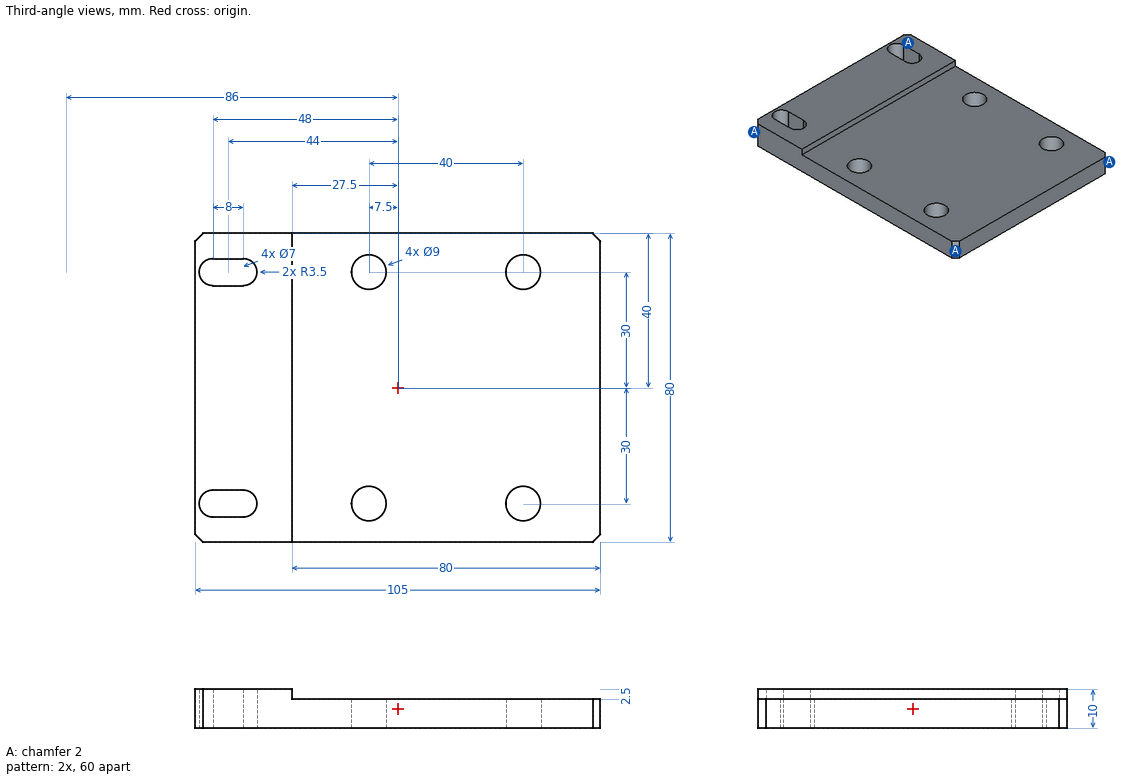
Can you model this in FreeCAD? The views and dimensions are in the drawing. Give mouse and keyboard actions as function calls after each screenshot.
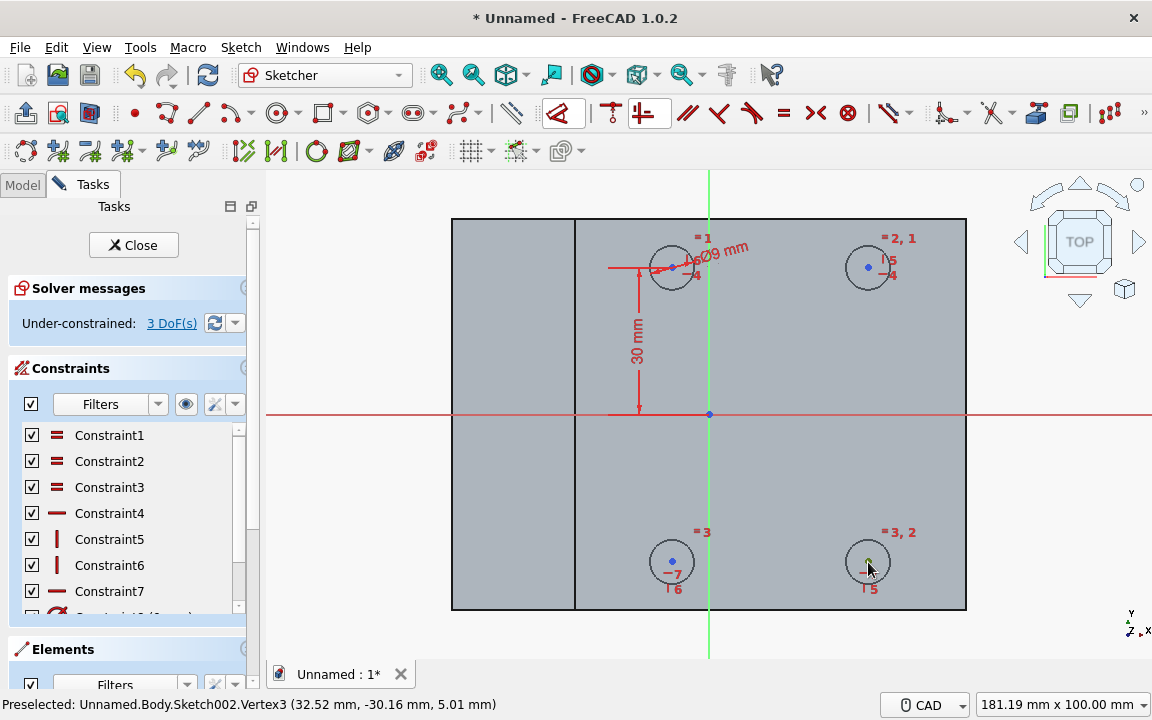
click(580, 114)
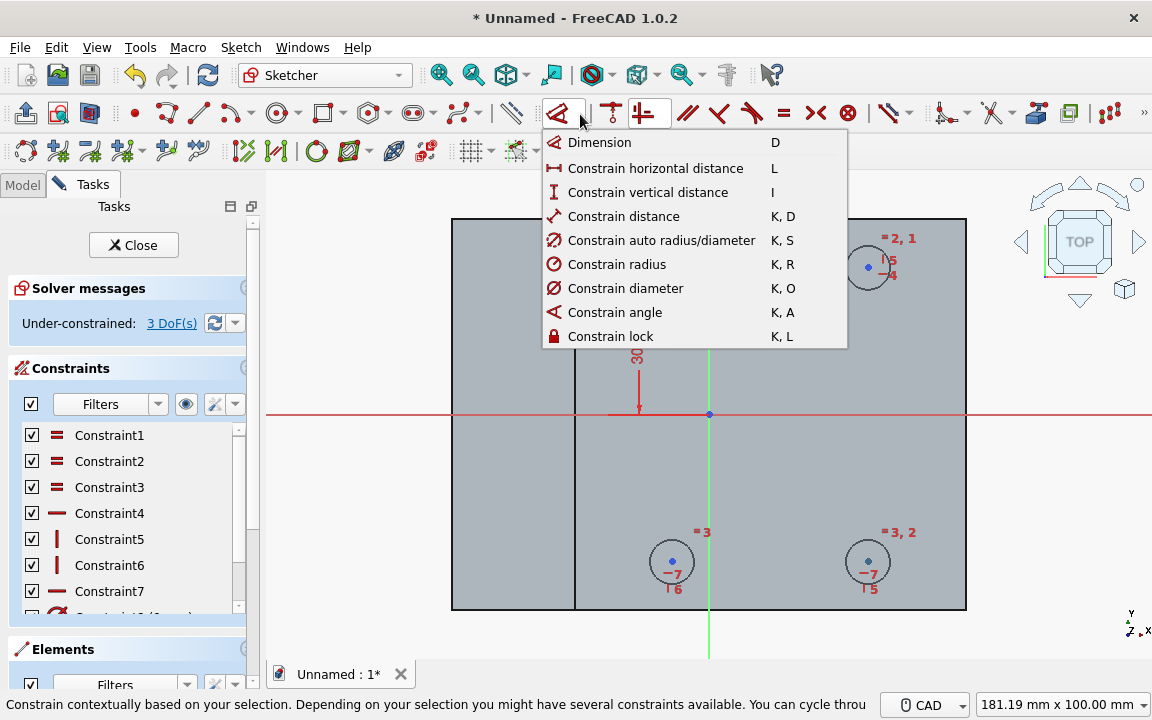
click(695, 192)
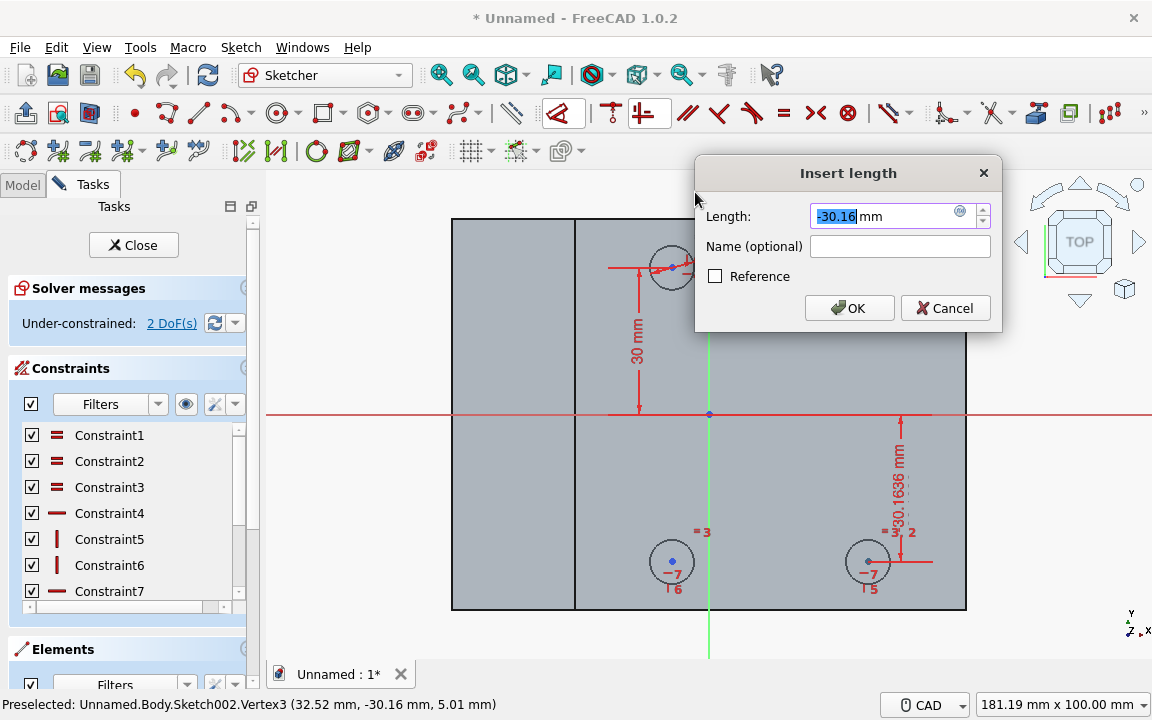
text(-30)
key(Return)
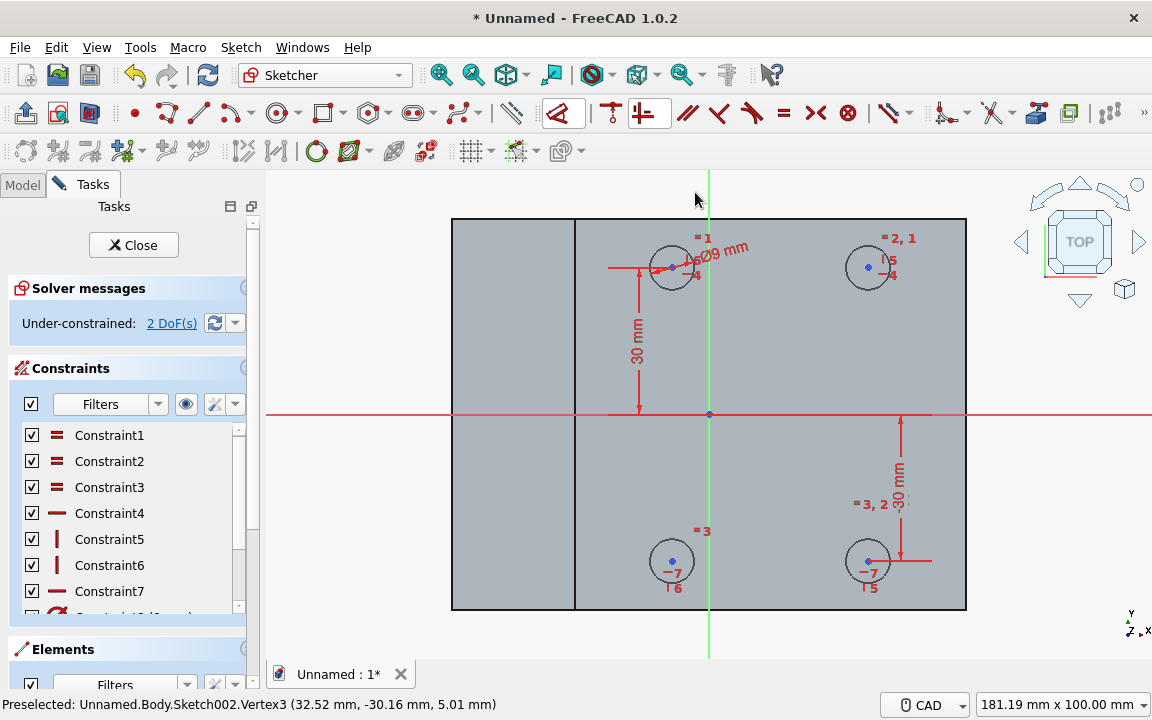
click(672, 268)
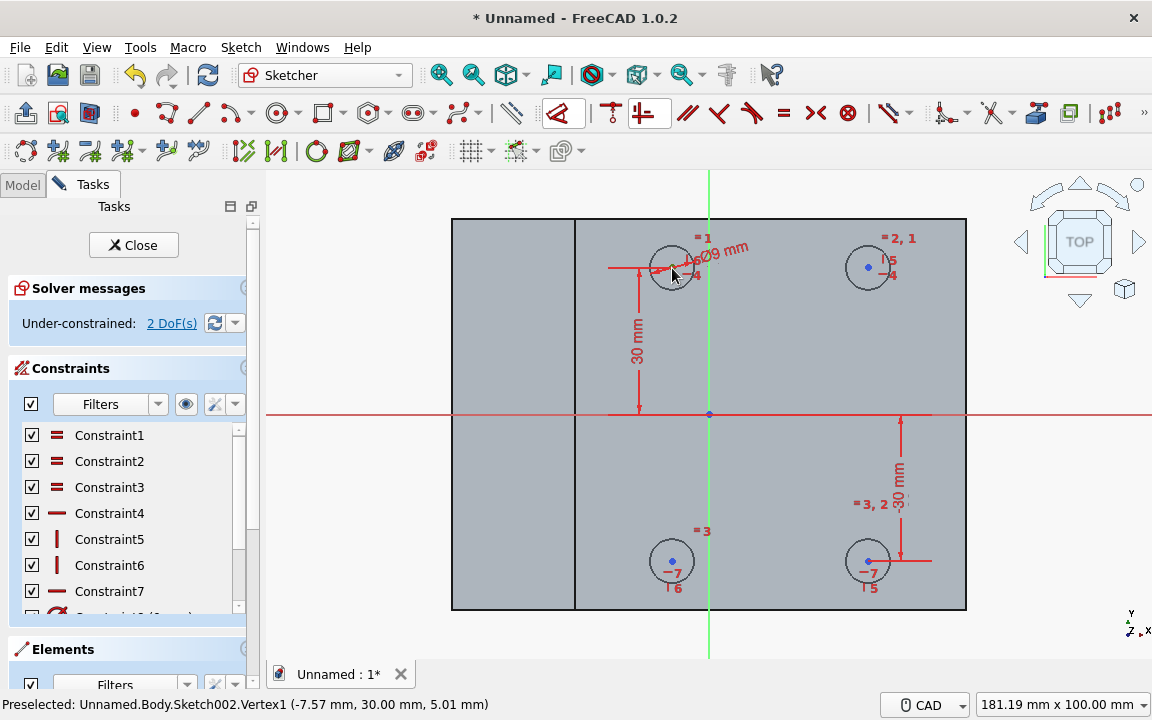
click(580, 114)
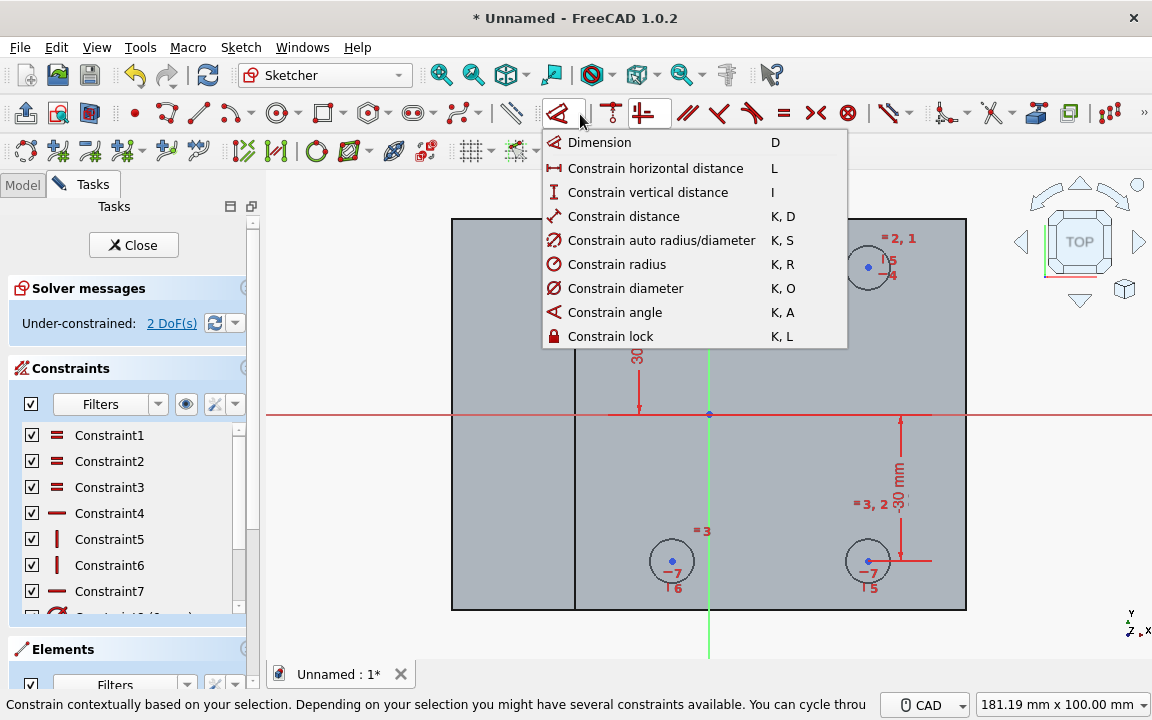
click(695, 168)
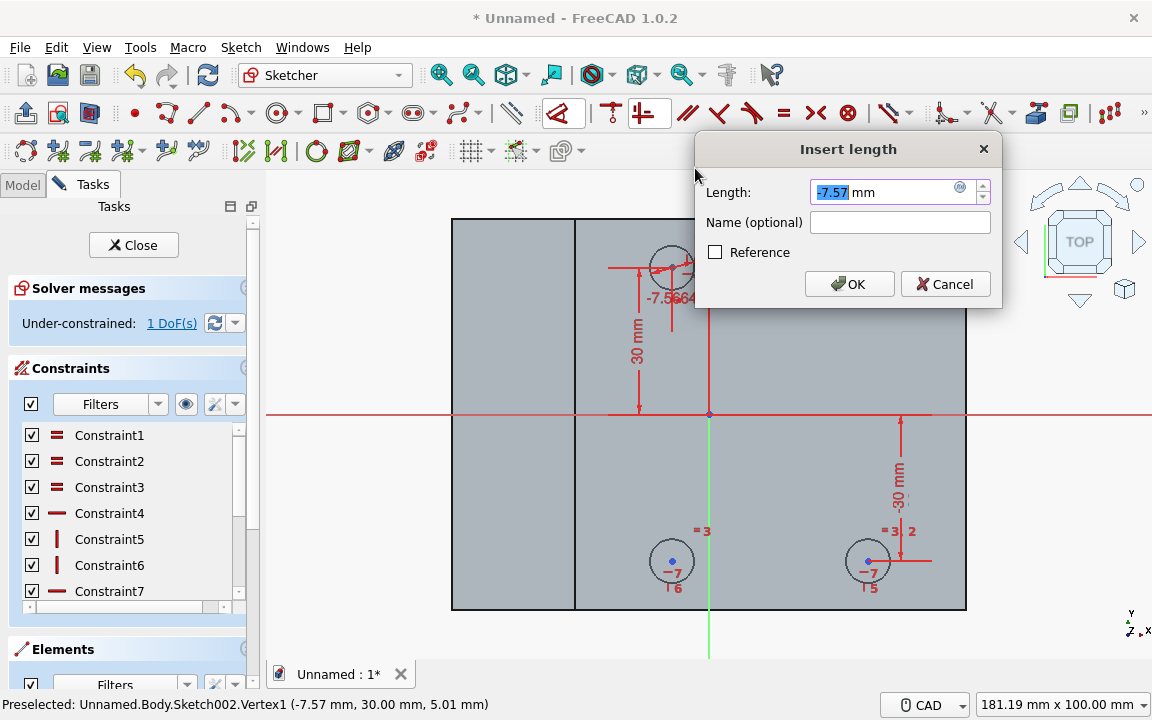
text(-7.5)
key(Return)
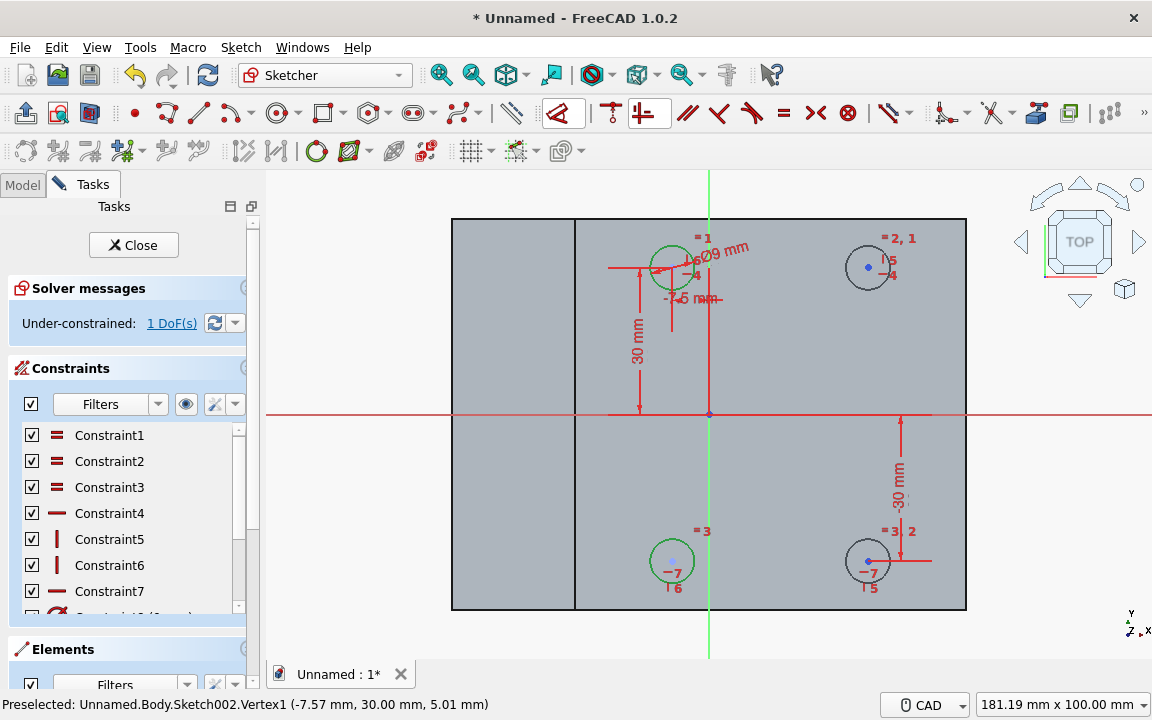
click(672, 268)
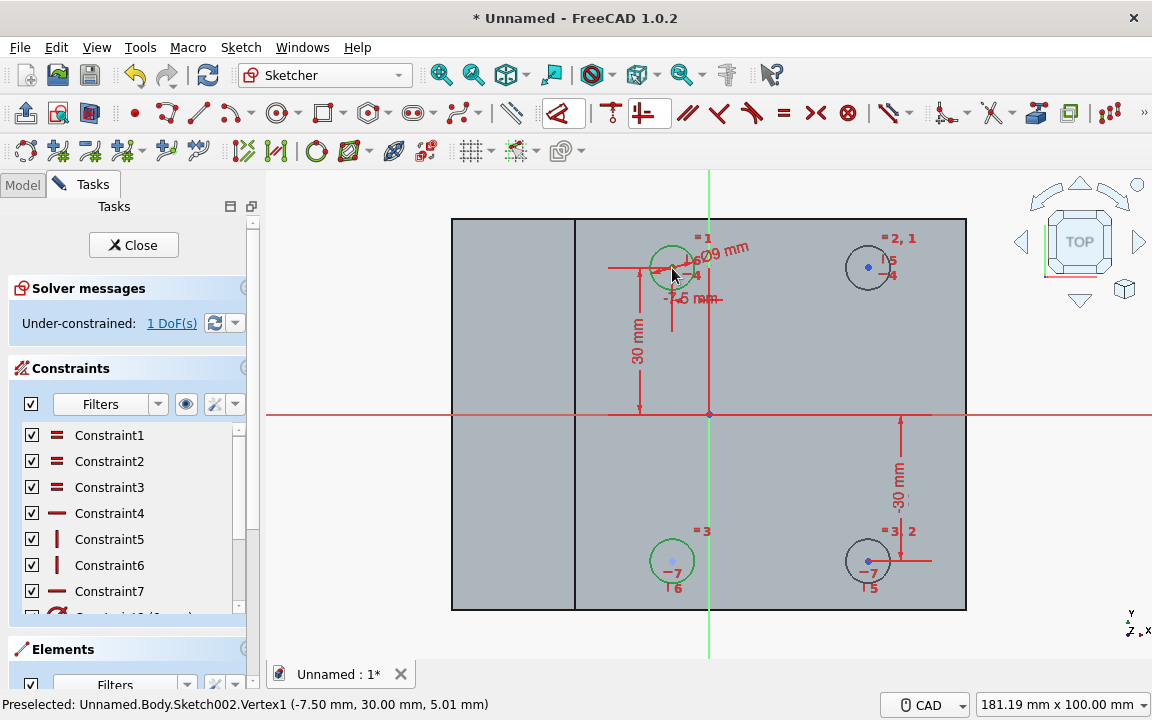
click(868, 268)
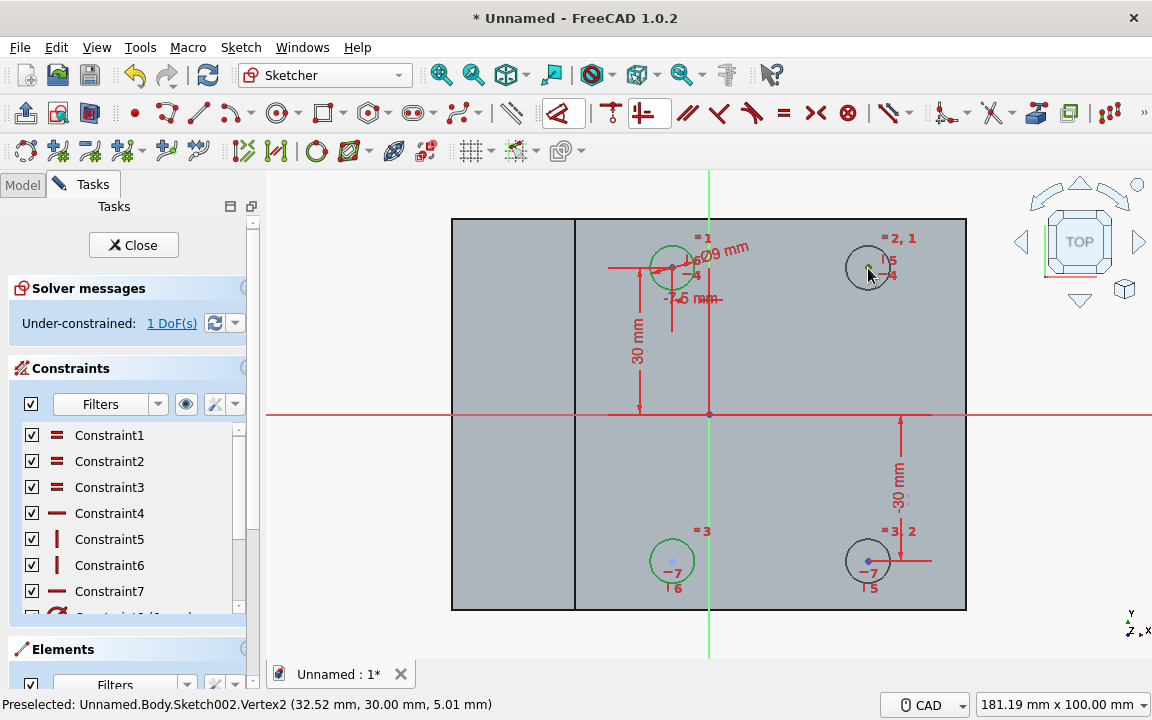
key(l)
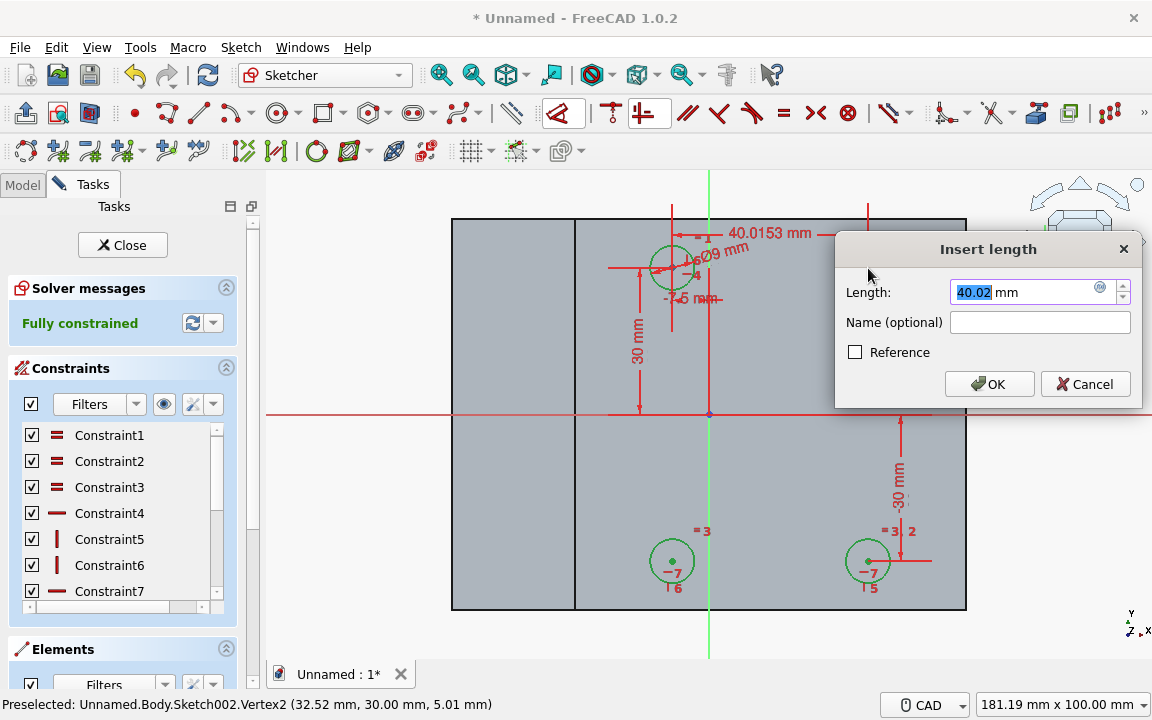
text(40)
key(Return)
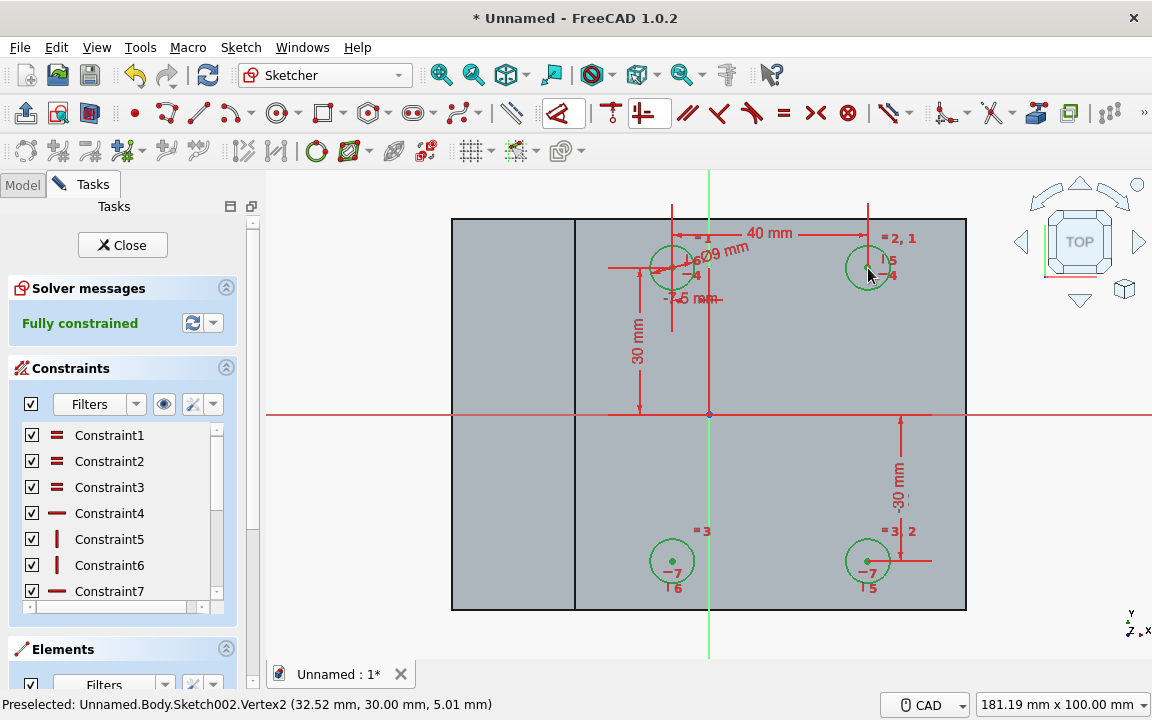
click(123, 245)